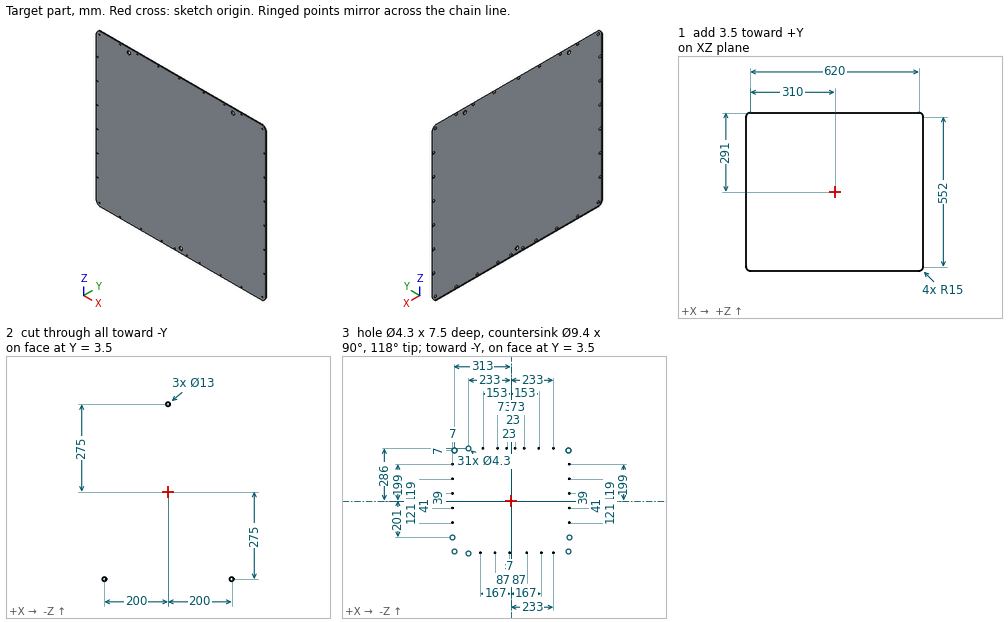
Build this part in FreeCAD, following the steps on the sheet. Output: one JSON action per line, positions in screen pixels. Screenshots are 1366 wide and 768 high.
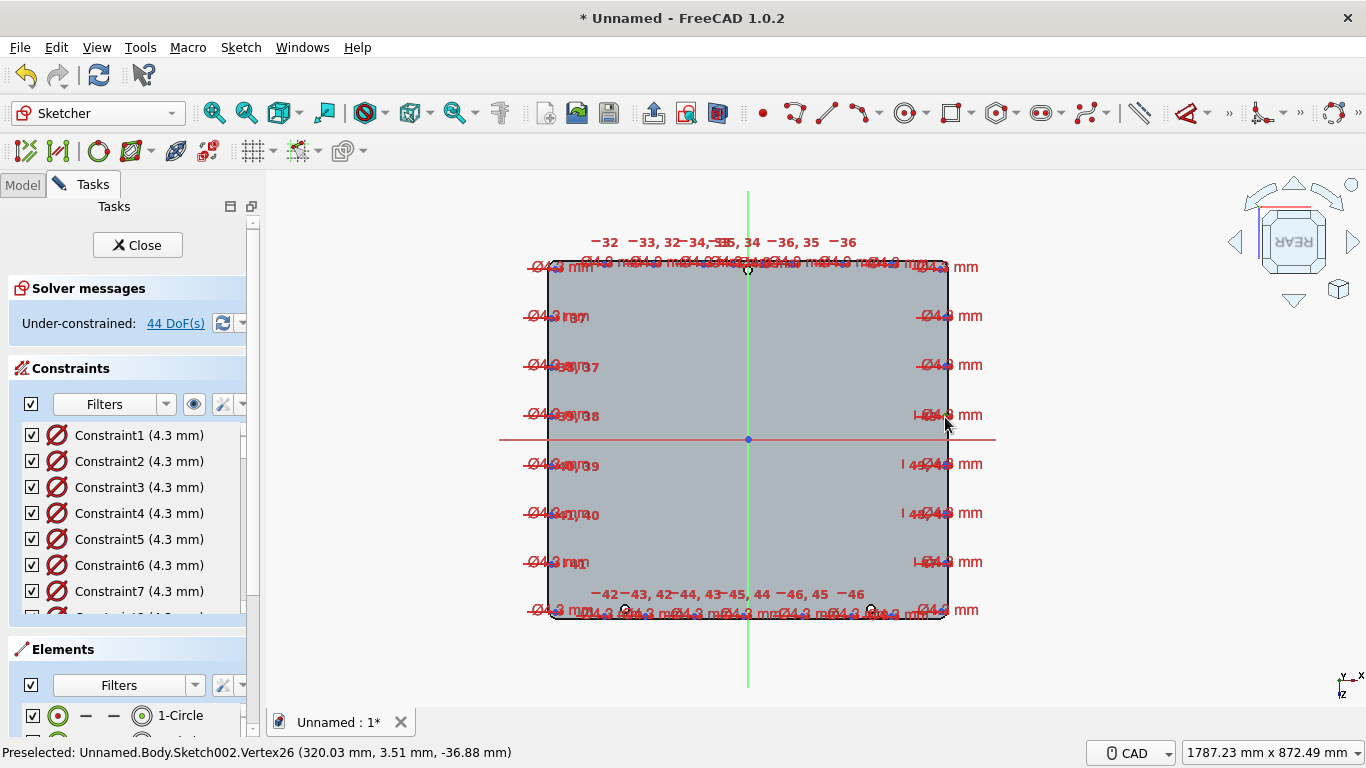
{"action": "left_click", "coordinate": [945, 367]}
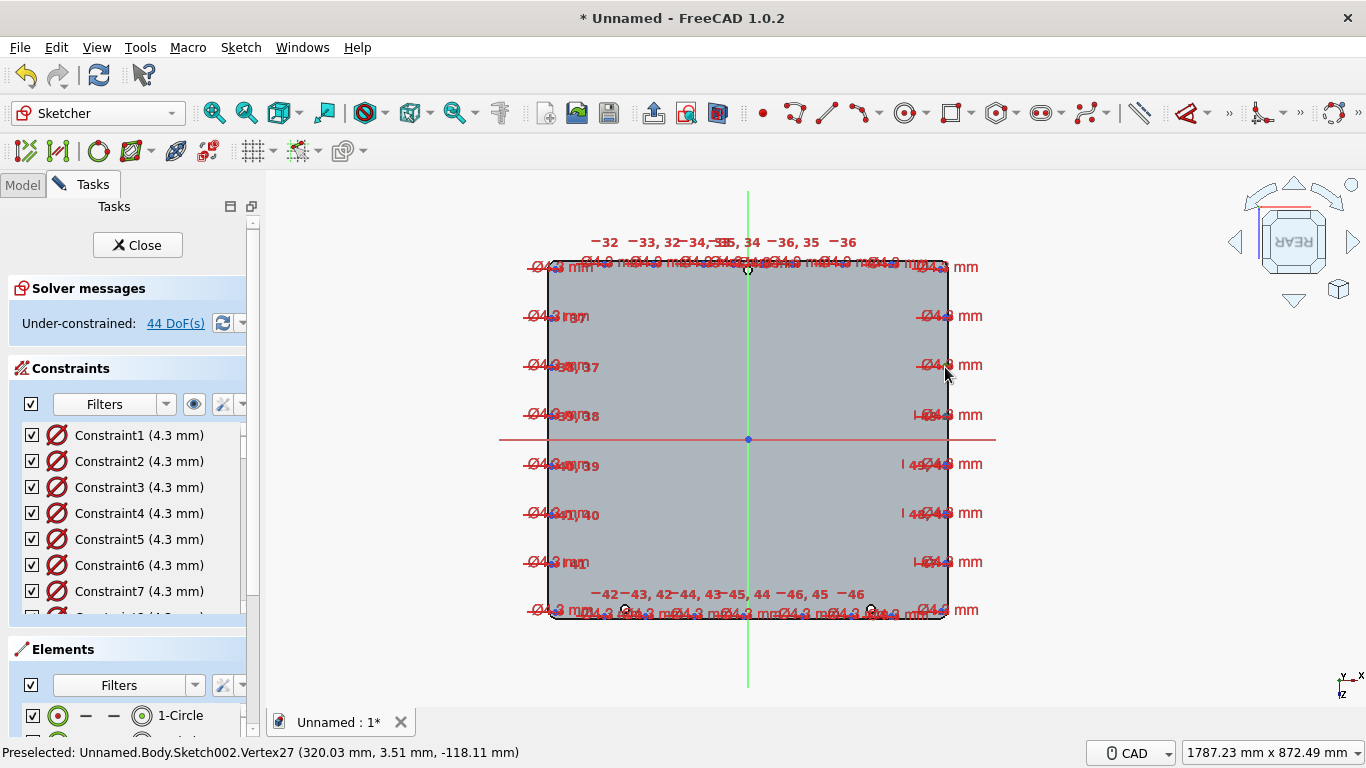
{"action": "key", "text": "v"}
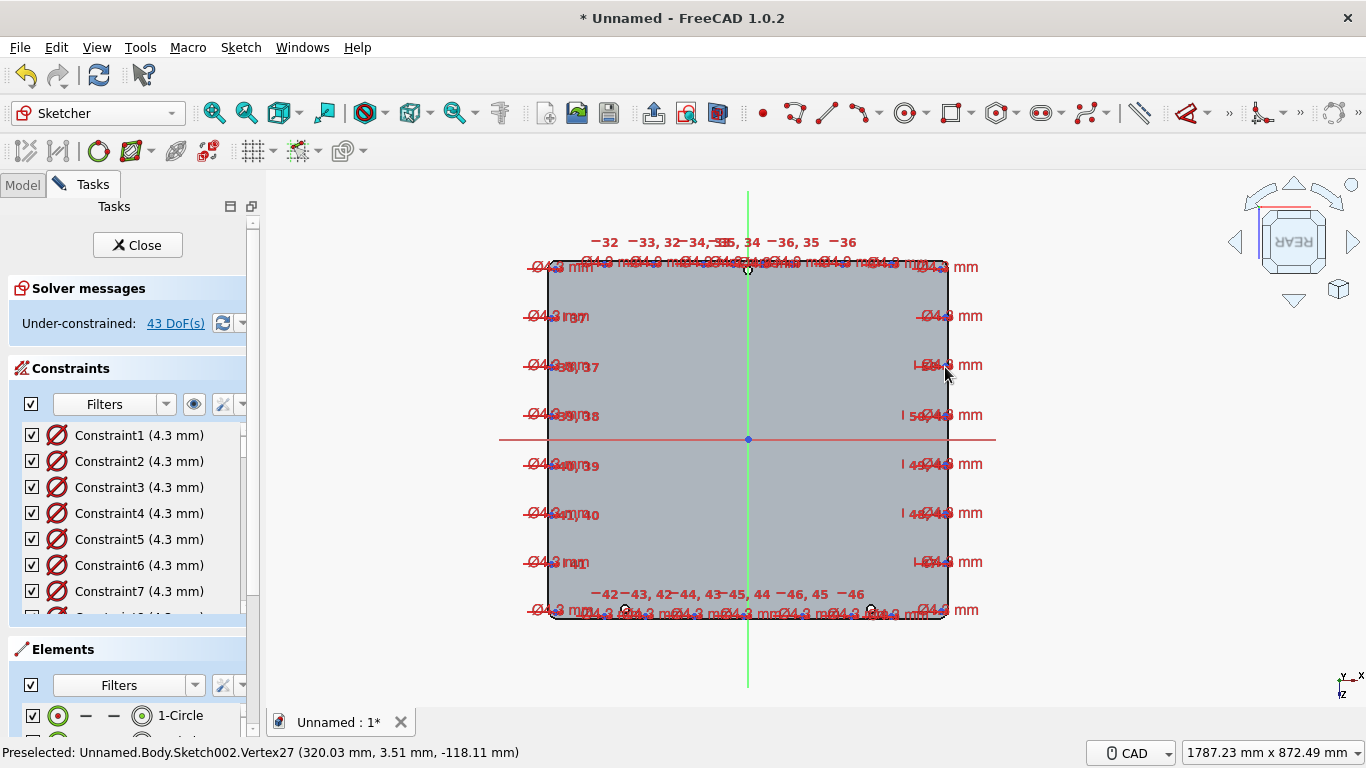
{"action": "left_click", "coordinate": [945, 367]}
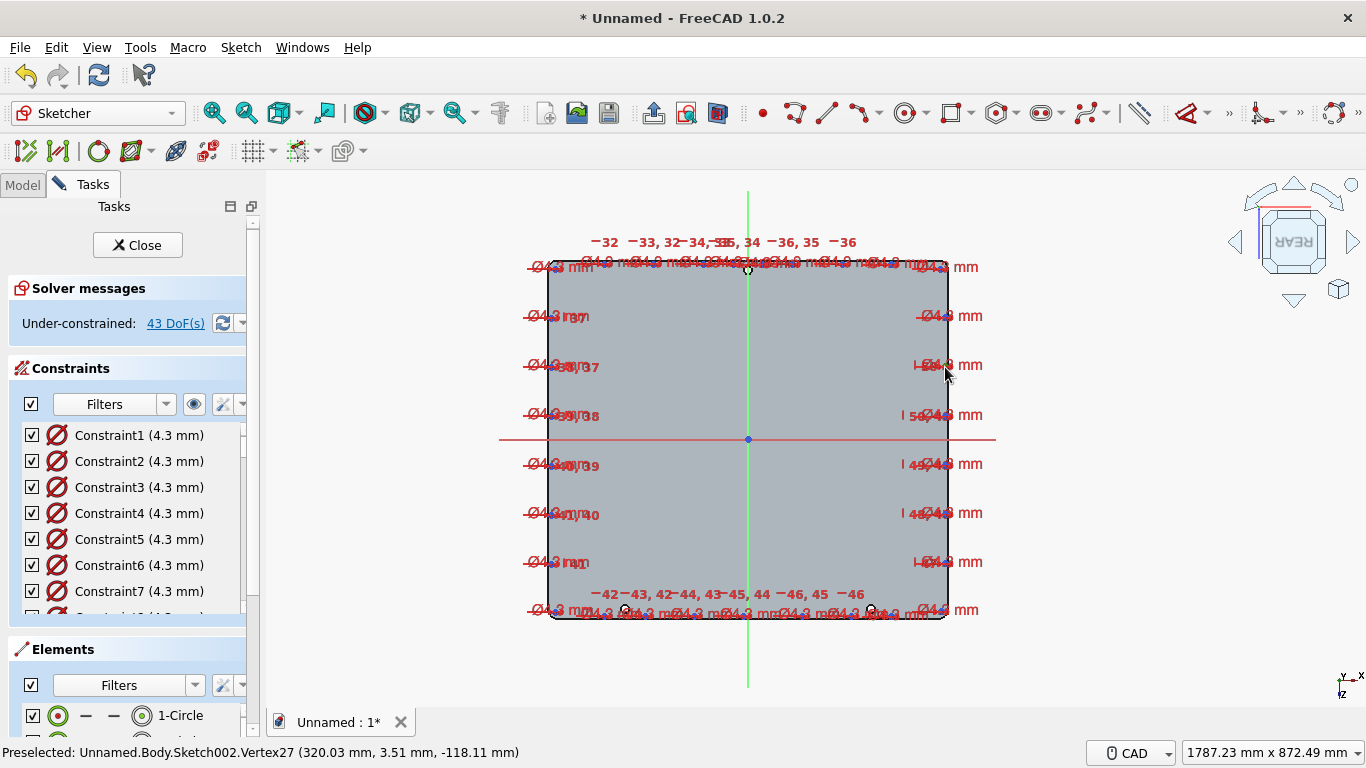
{"action": "left_click", "coordinate": [945, 318]}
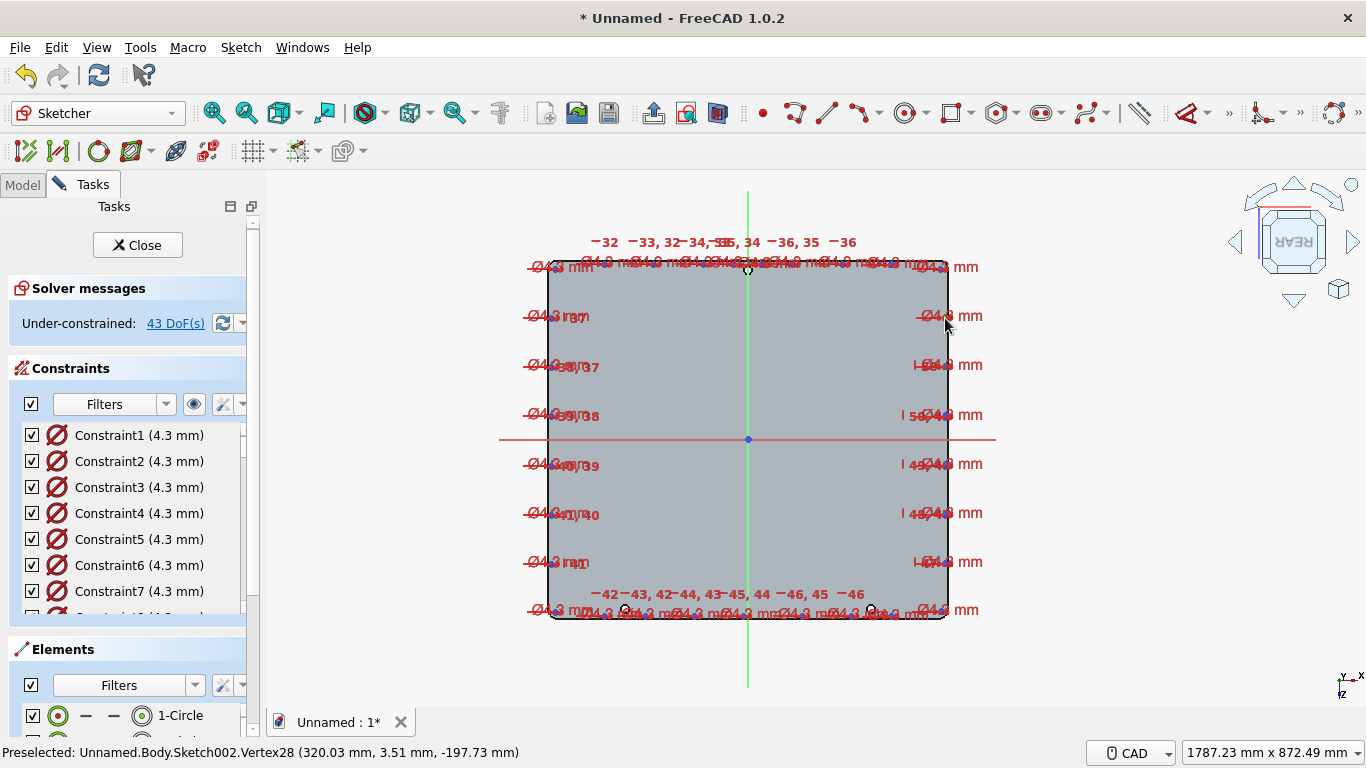
{"action": "key", "text": "v"}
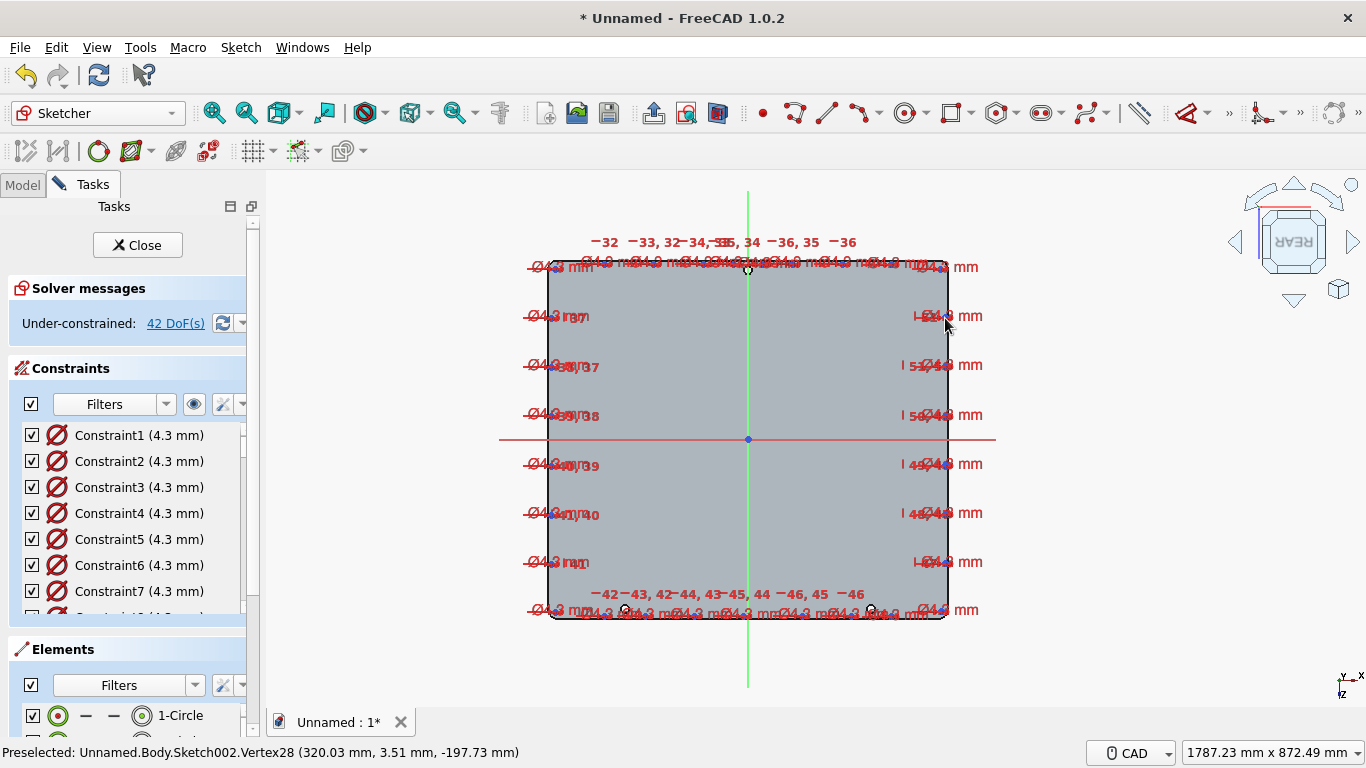
{"action": "left_click", "coordinate": [843, 264]}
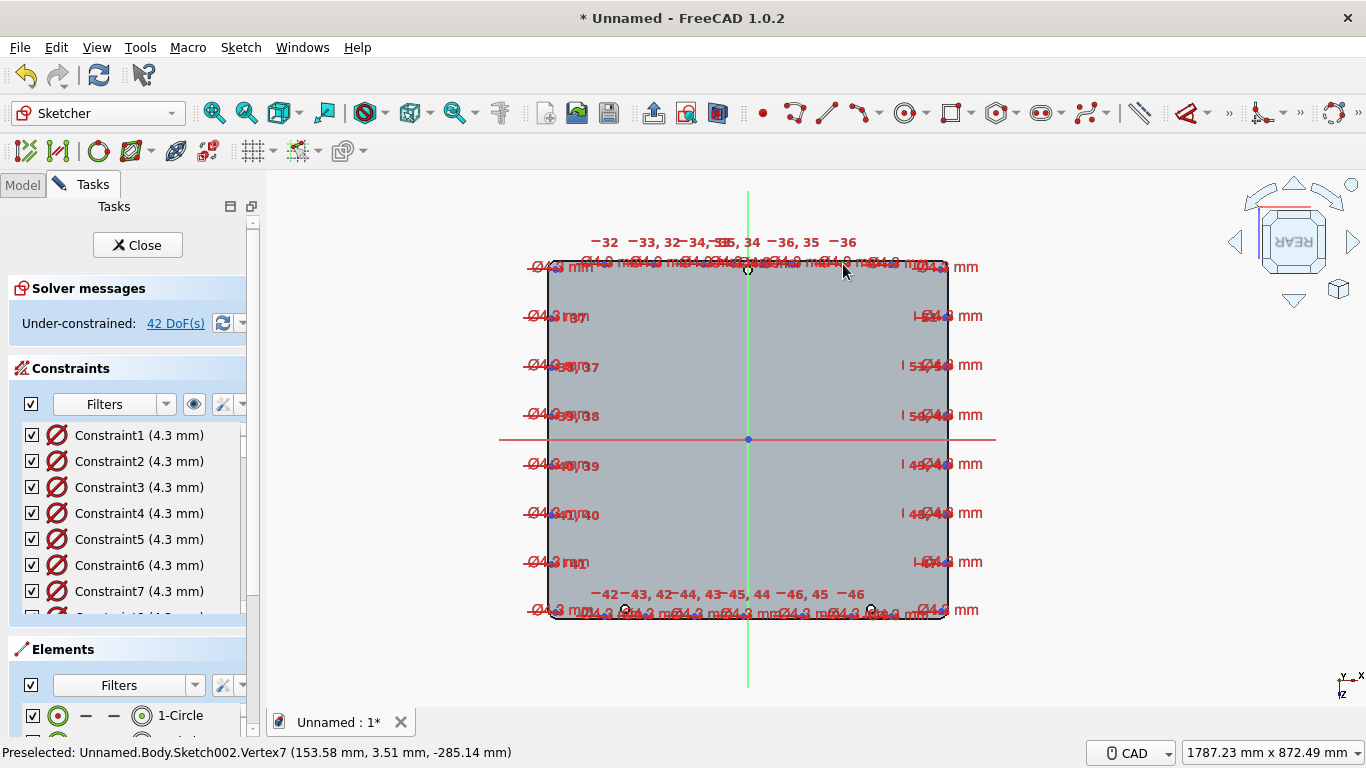
{"action": "left_click", "coordinate": [891, 265]}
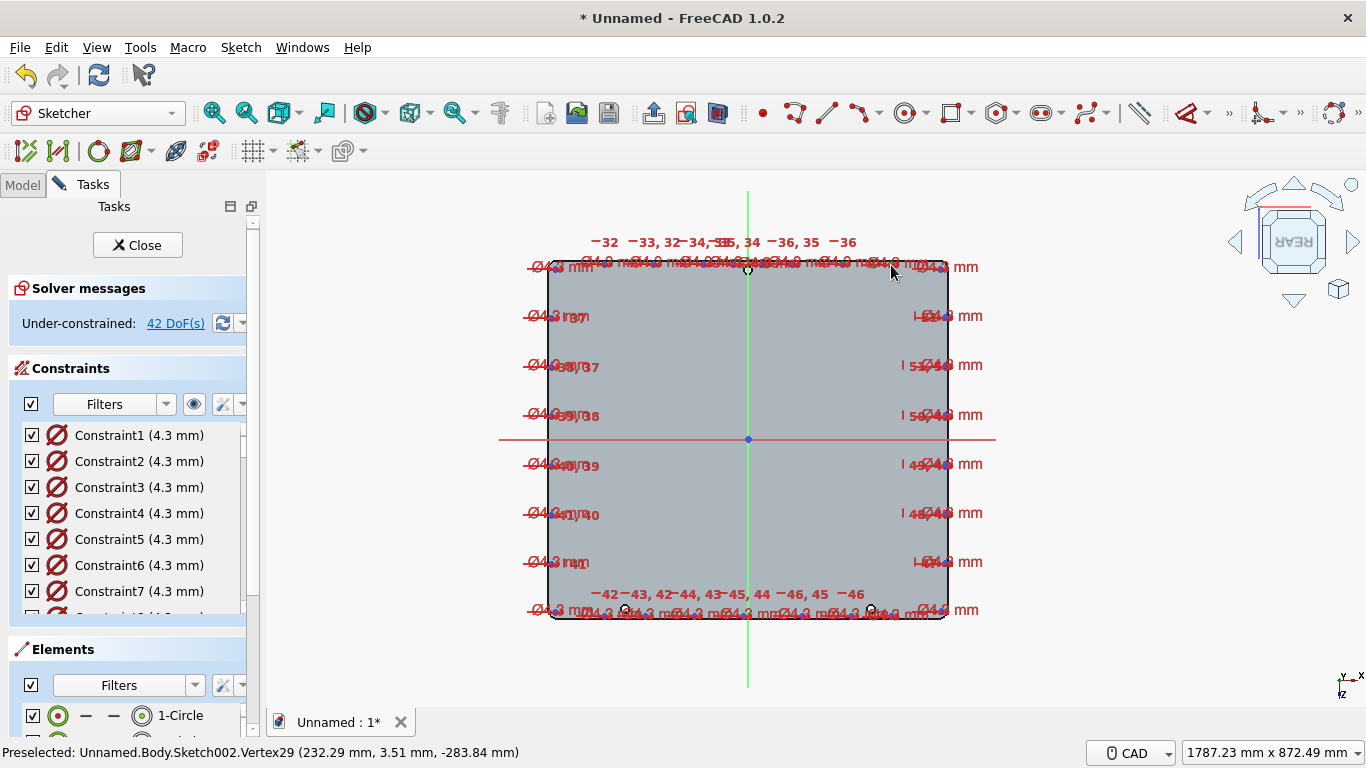
{"action": "key", "text": "h"}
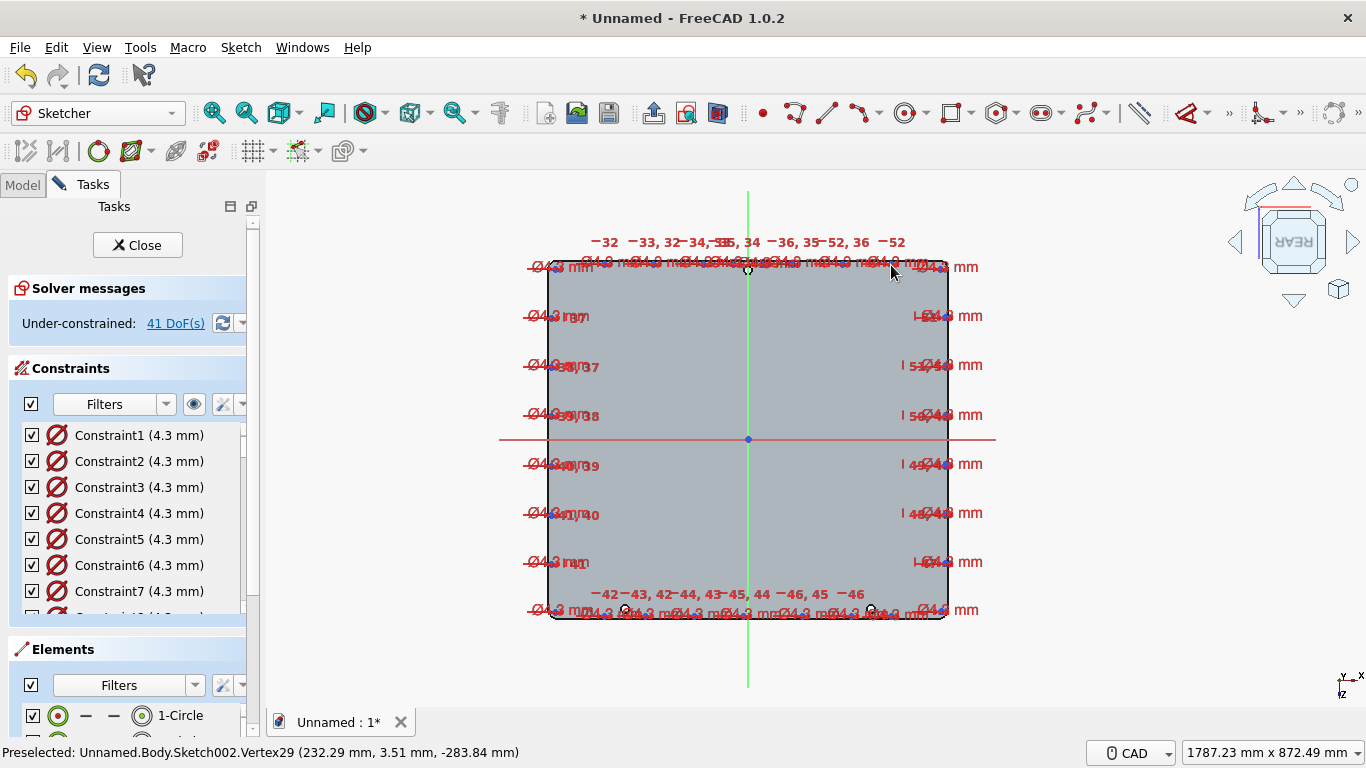
{"action": "left_click", "coordinate": [734, 264]}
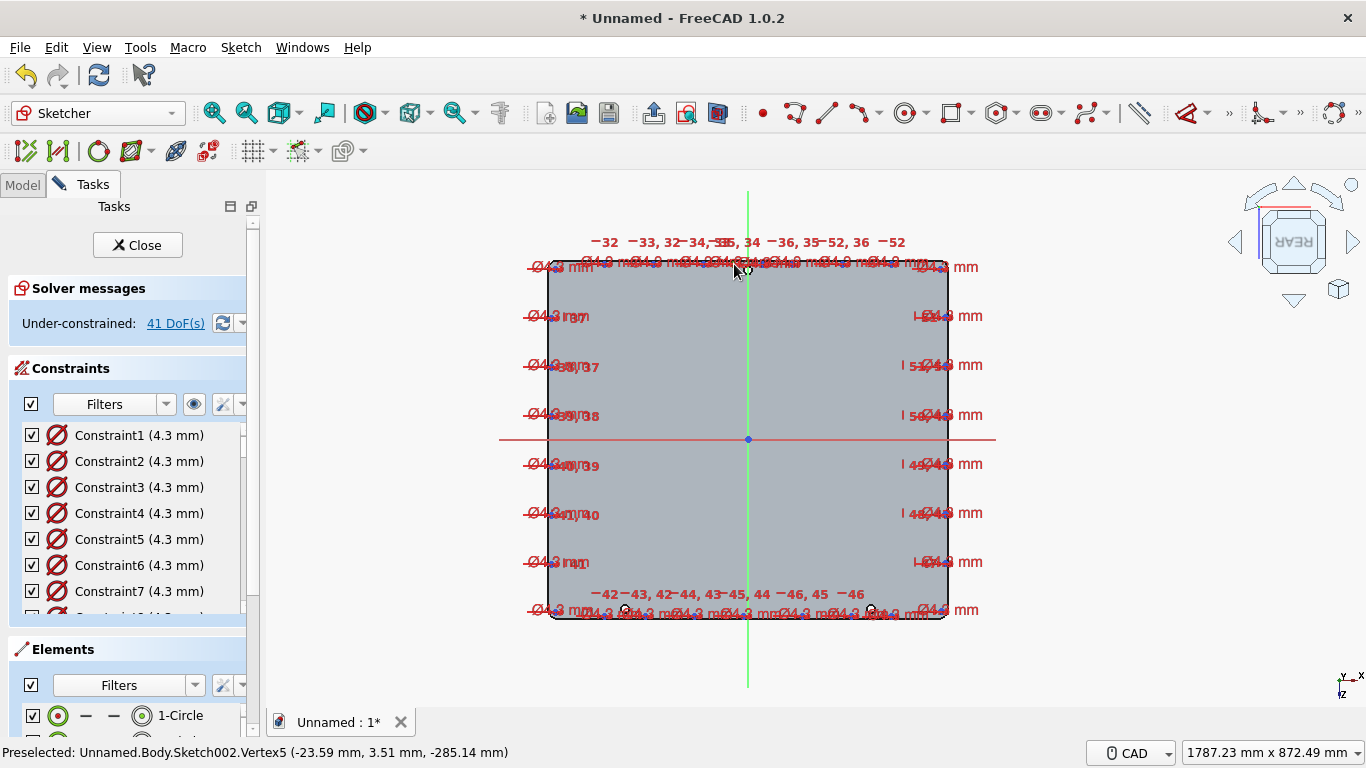
{"action": "left_click", "coordinate": [762, 265]}